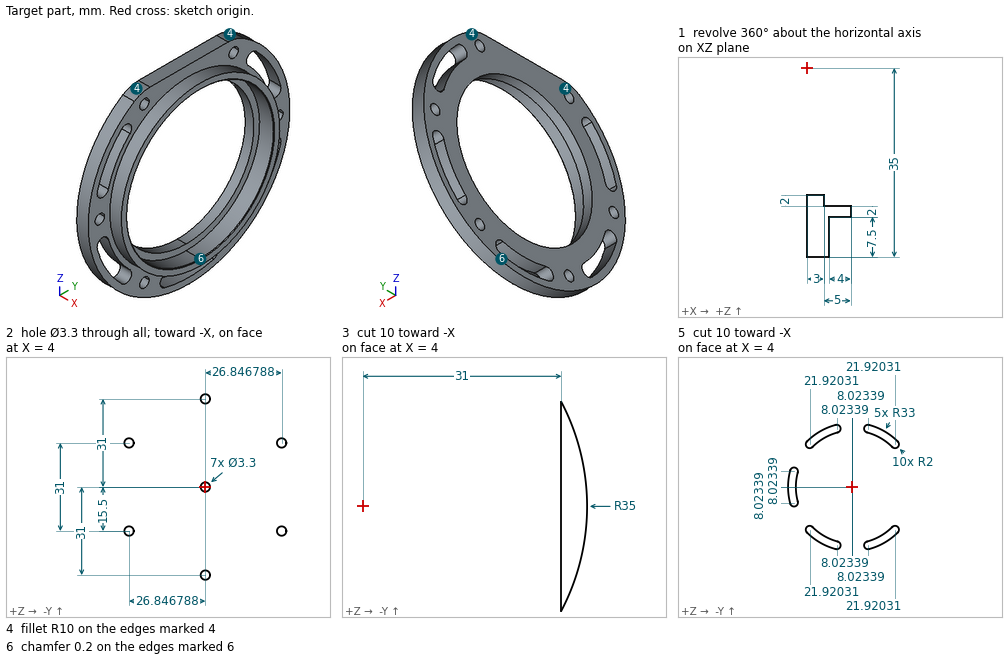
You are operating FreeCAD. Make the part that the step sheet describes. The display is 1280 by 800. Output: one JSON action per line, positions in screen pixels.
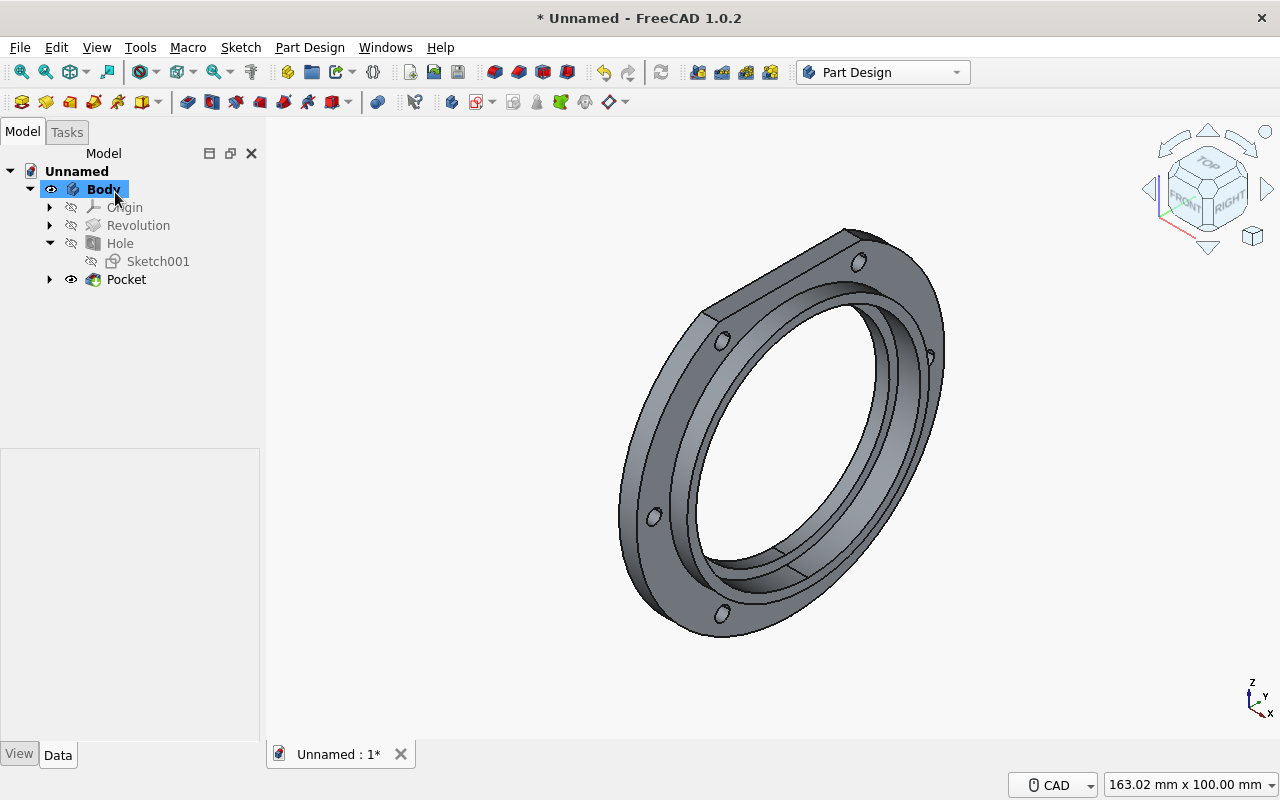
{"action": "key", "text": "2"}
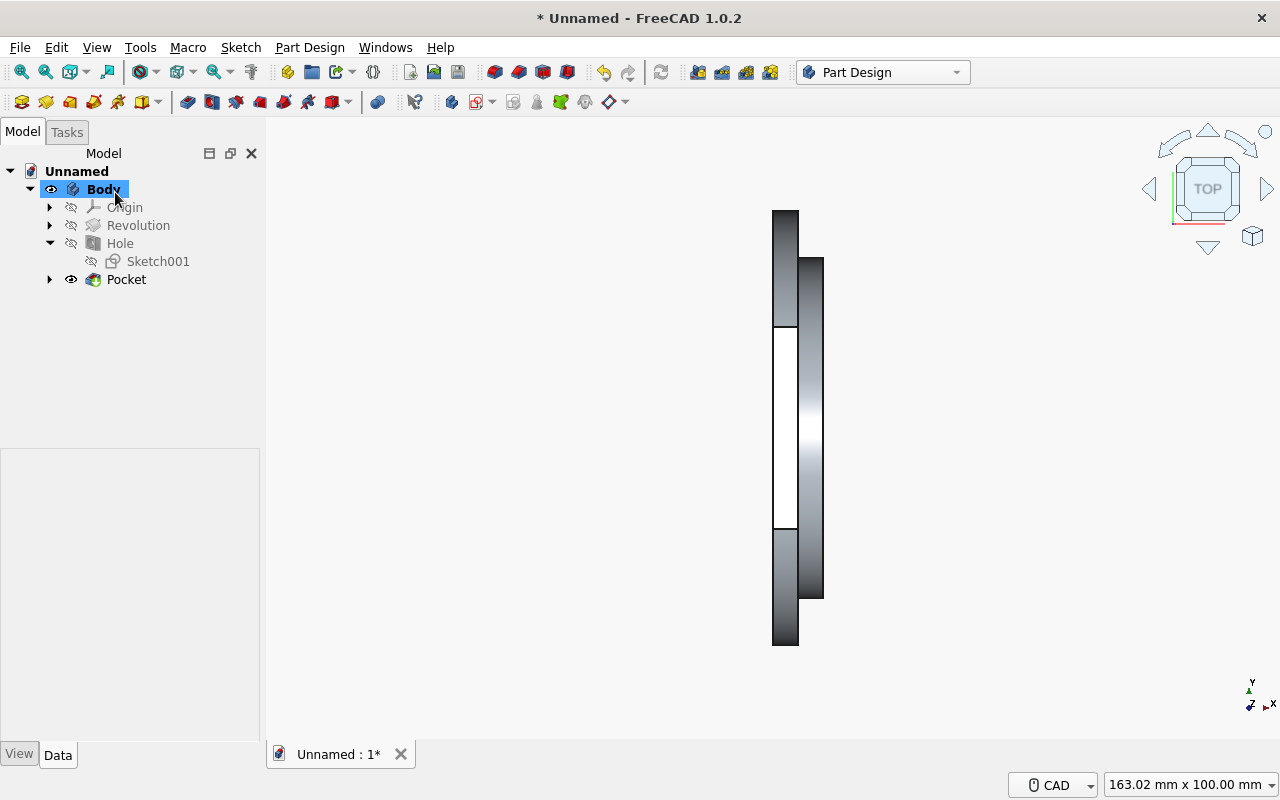
{"action": "left_click", "coordinate": [785, 326]}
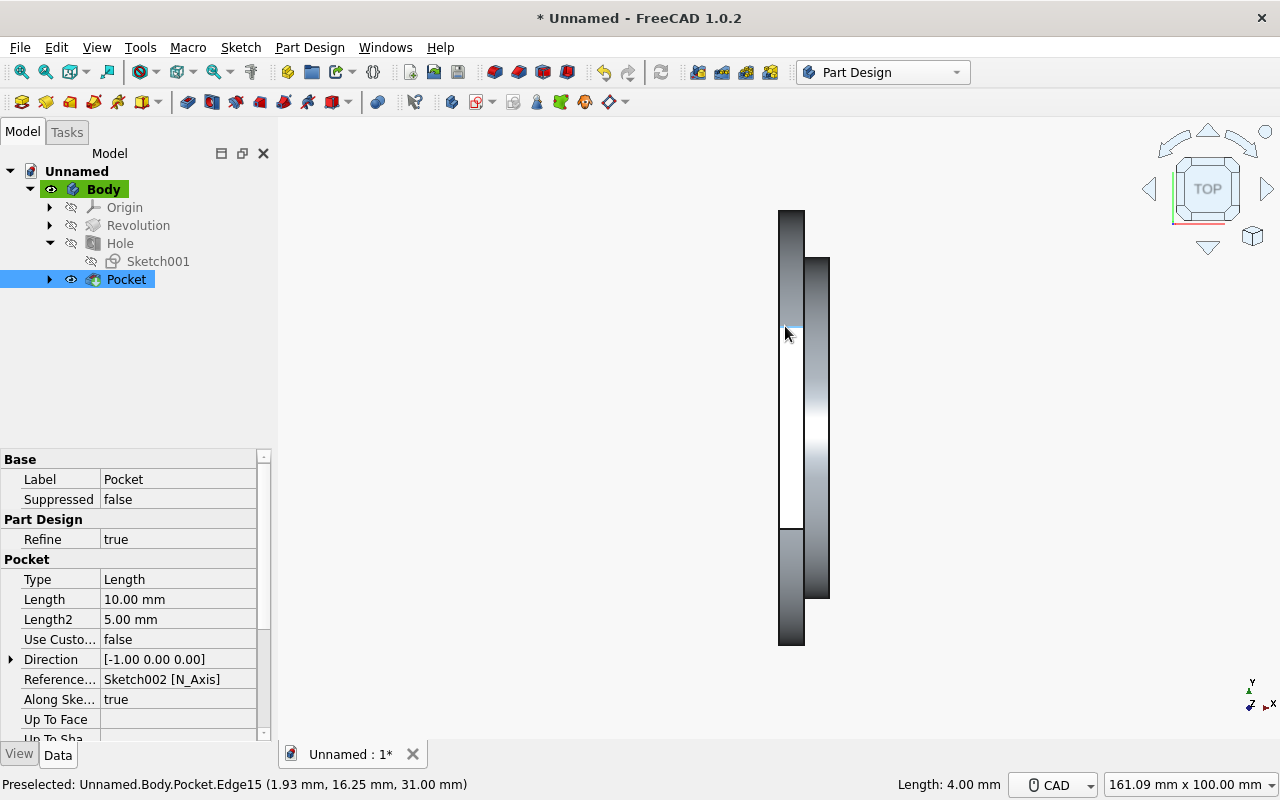
{"action": "key", "text": "1"}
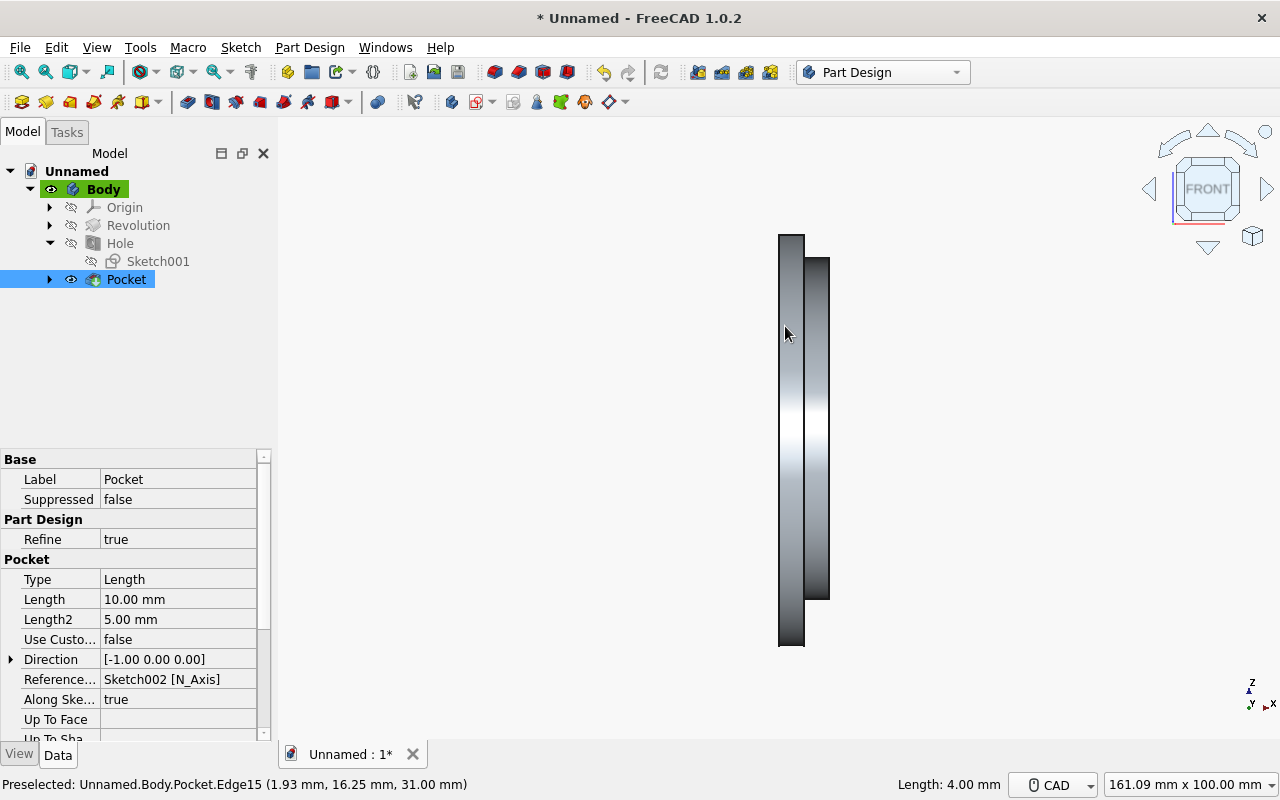
{"action": "key", "text": "3"}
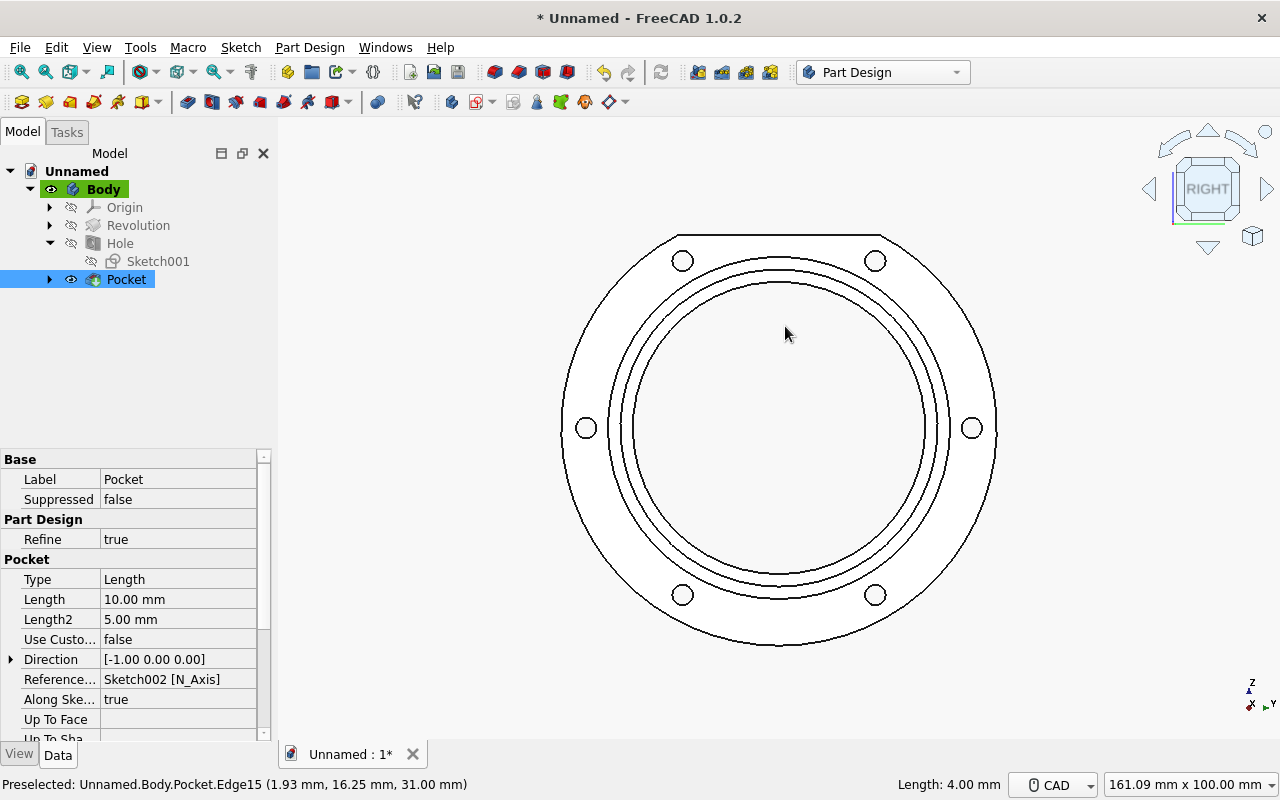
{"action": "key", "text": "5"}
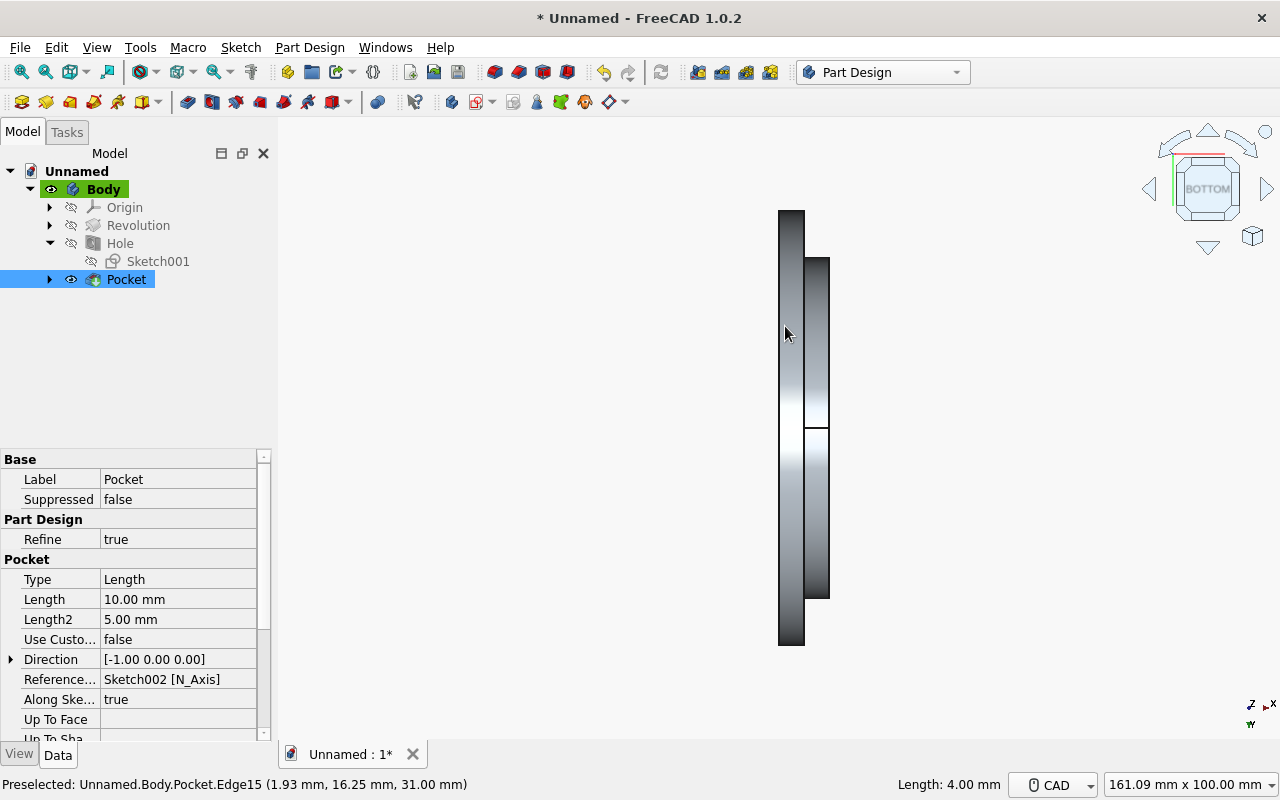
{"action": "key", "text": "4"}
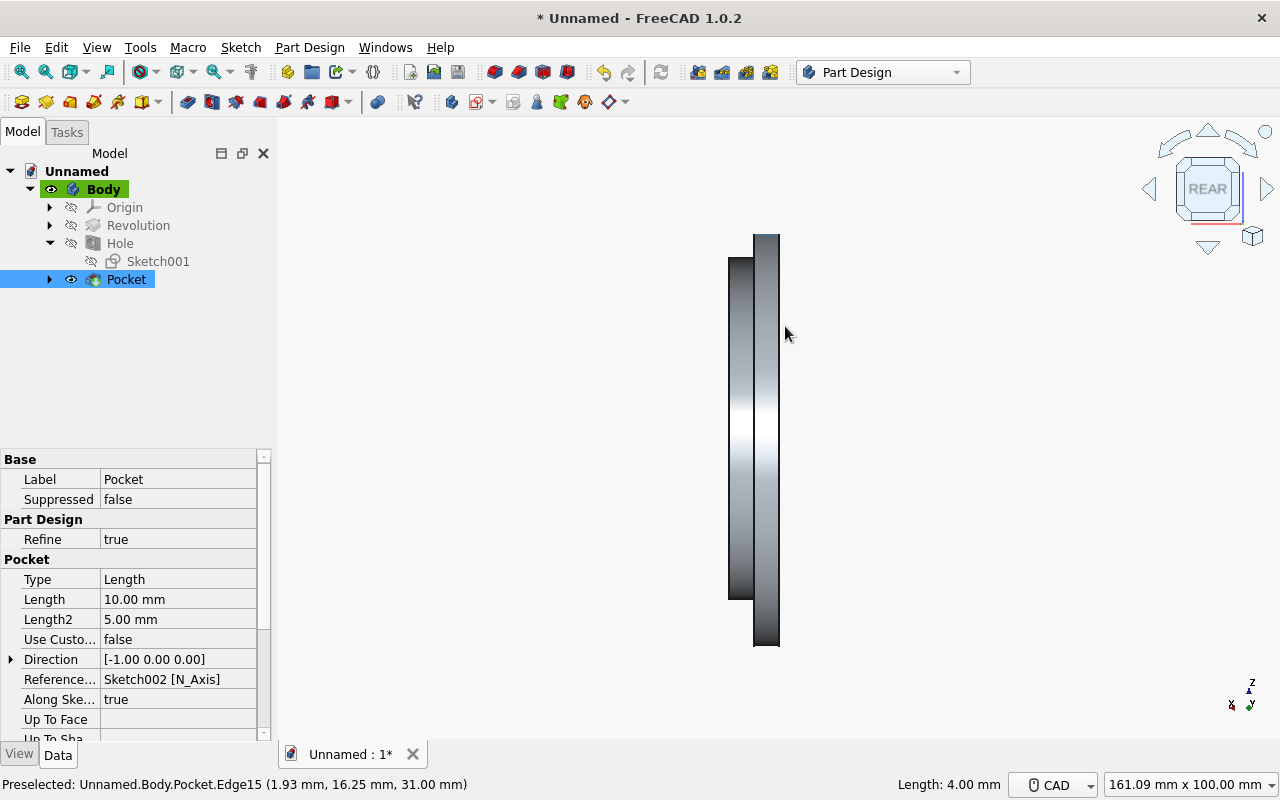
{"action": "key", "text": "6"}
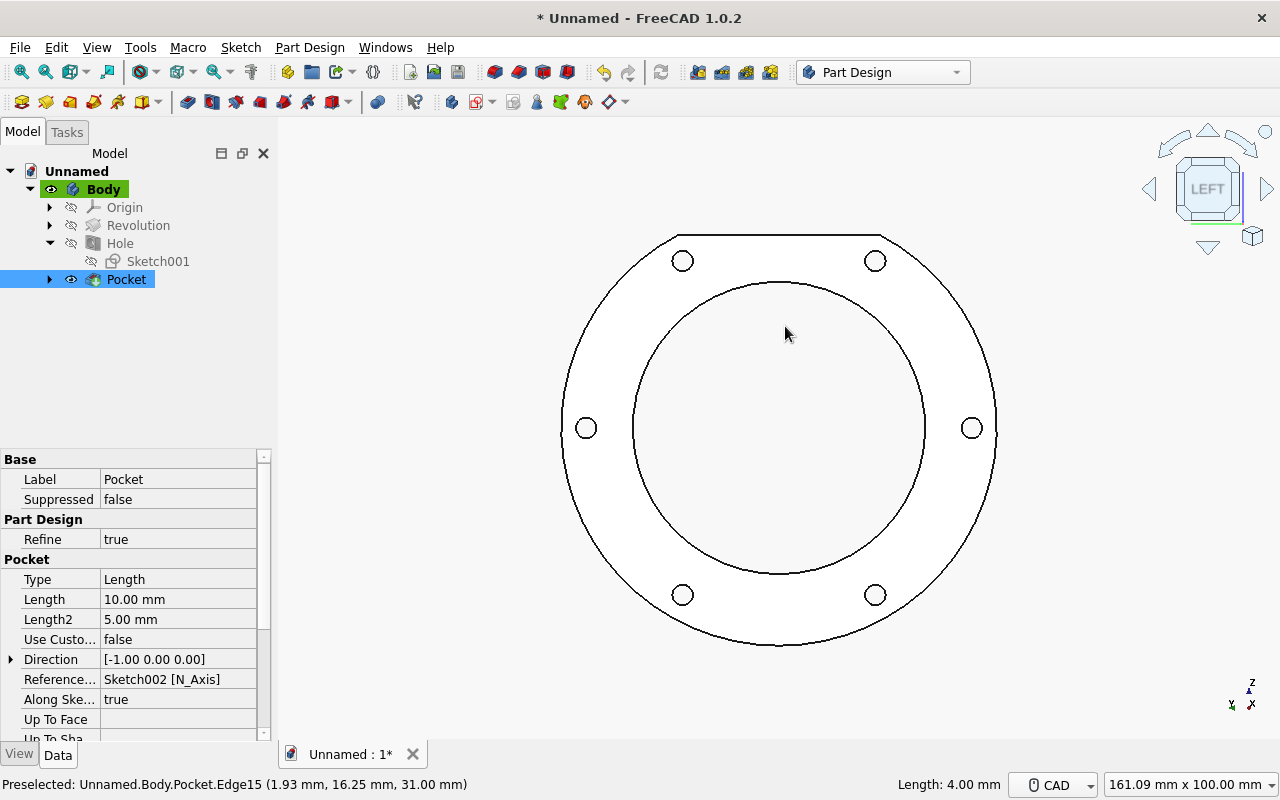
{"action": "key", "text": "v 3"}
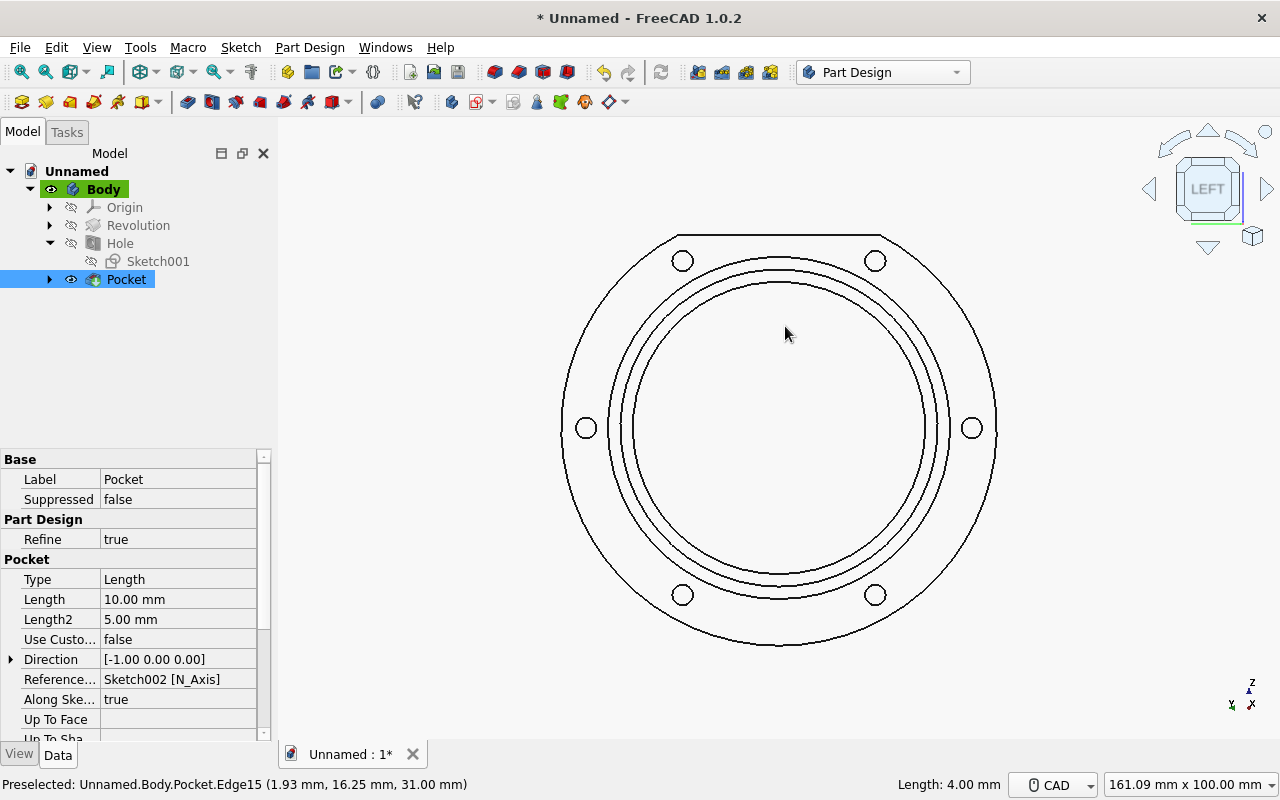
{"action": "key", "text": "0"}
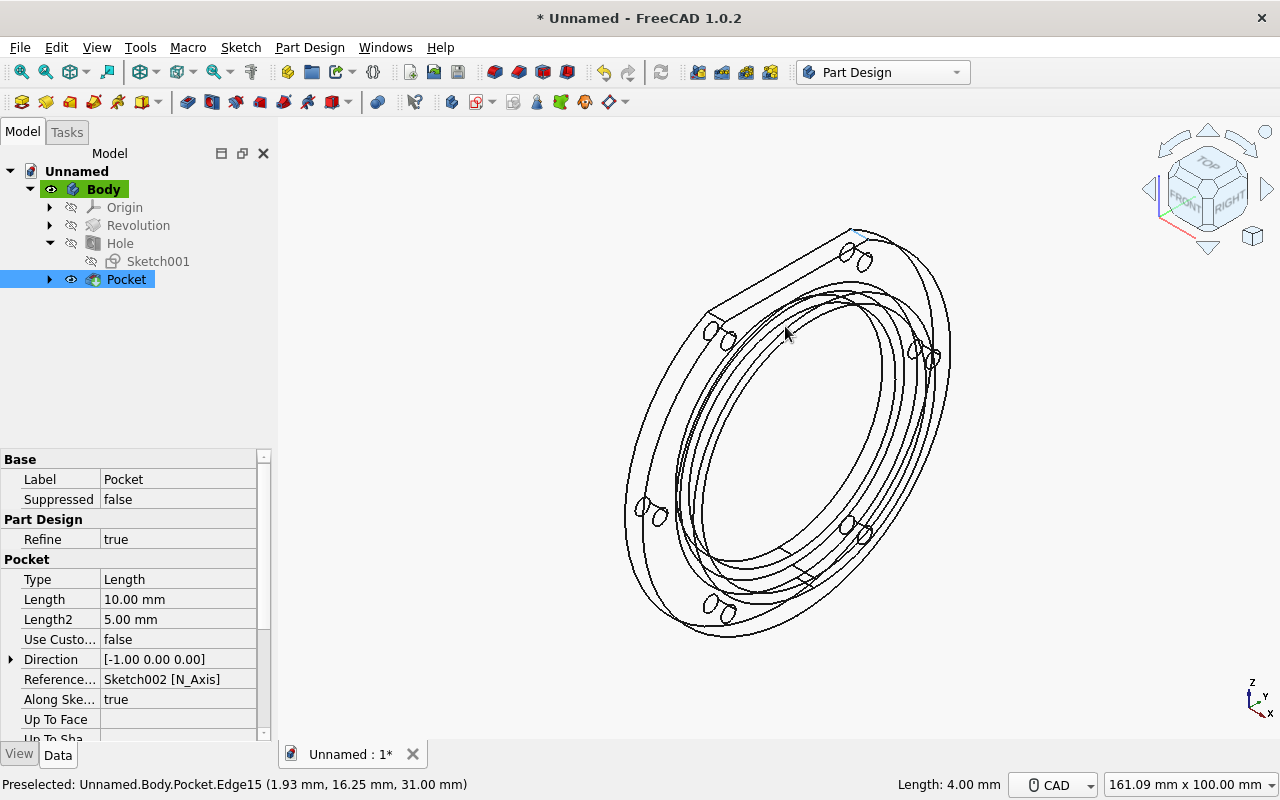
{"action": "left_click", "coordinate": [716, 316], "text": "ctrl"}